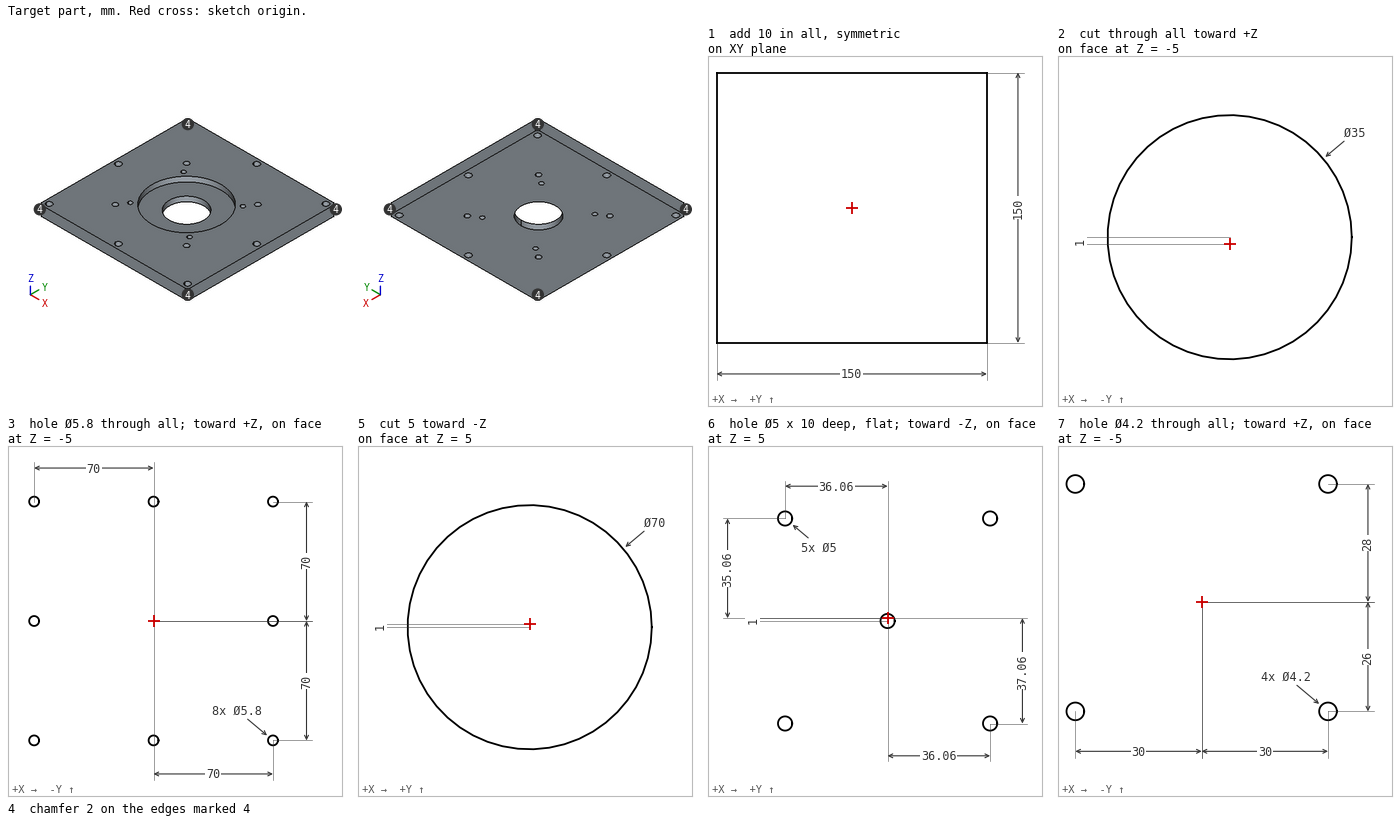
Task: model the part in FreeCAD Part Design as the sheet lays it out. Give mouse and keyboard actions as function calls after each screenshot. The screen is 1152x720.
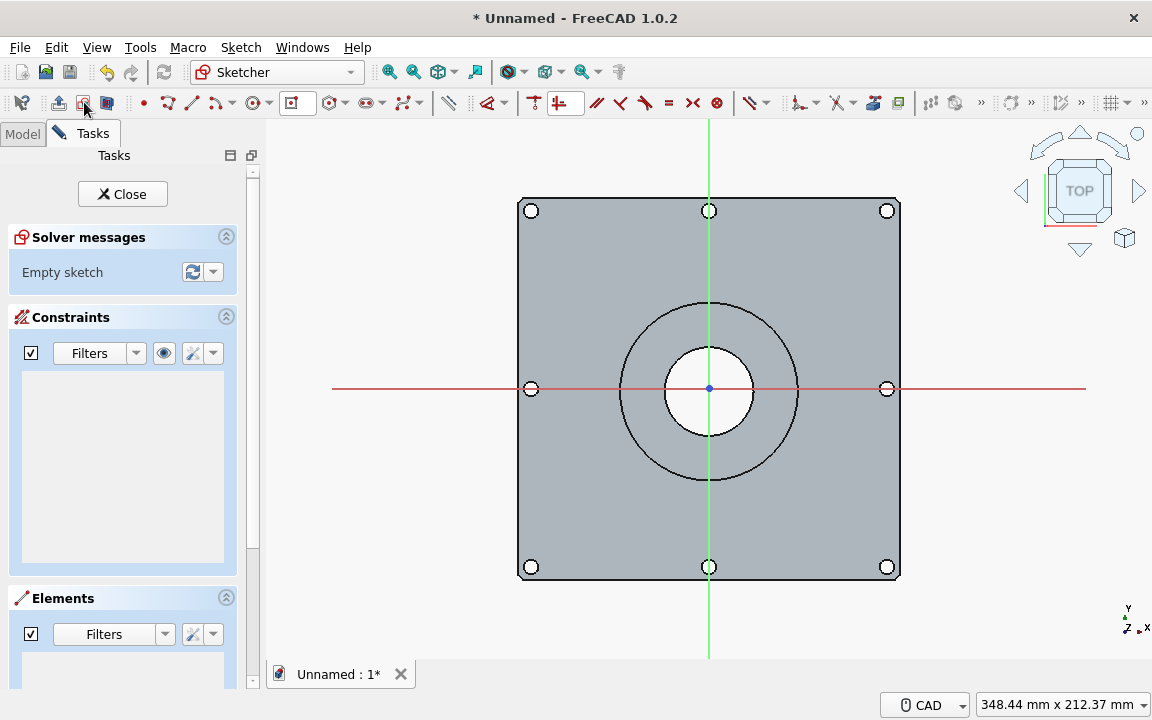
scroll(792, 395, up, 3)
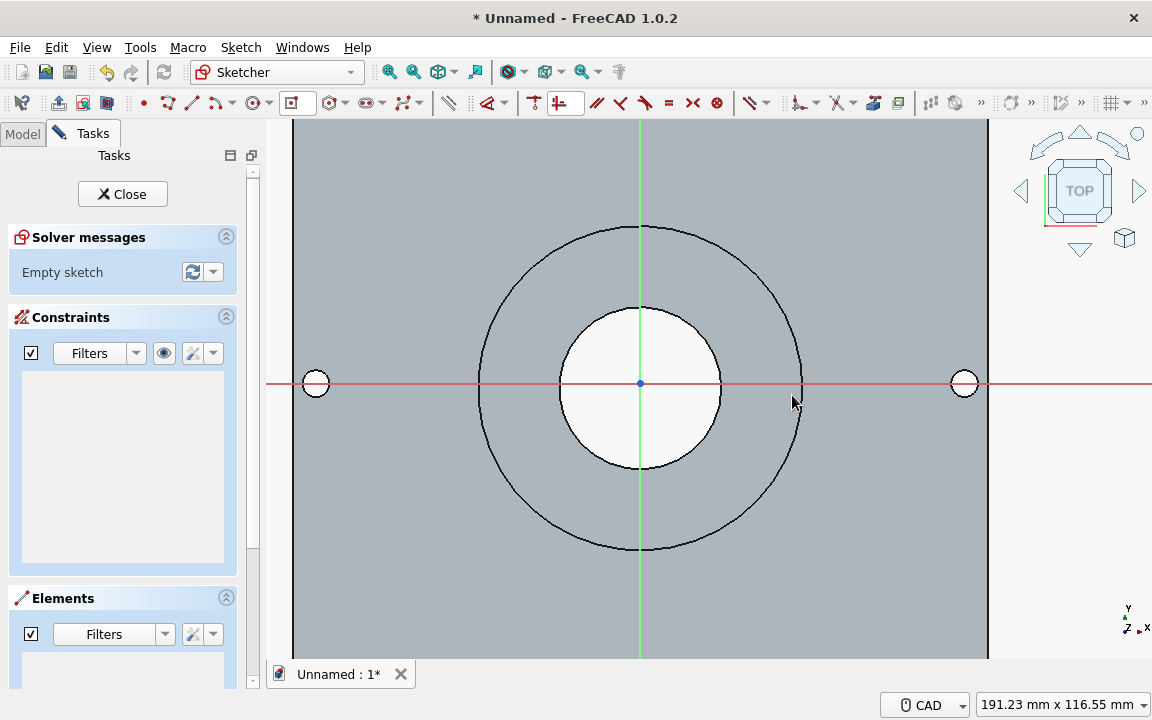
key(g)
key(c)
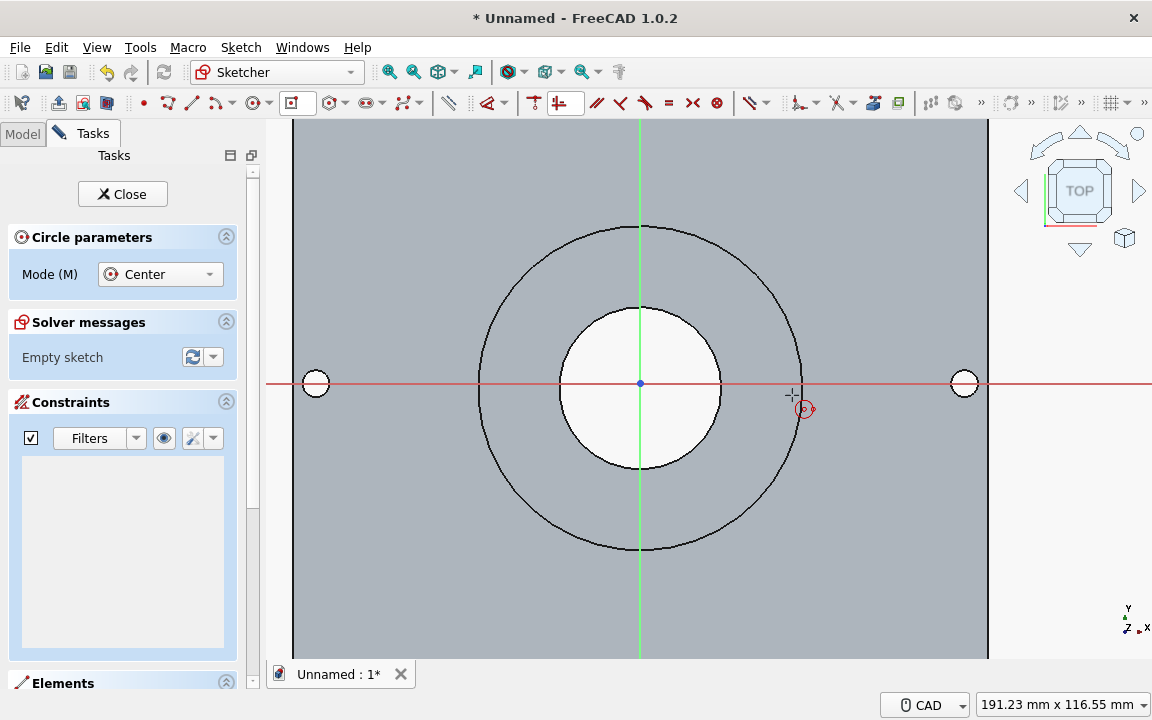
scroll(473, 221, up, 4)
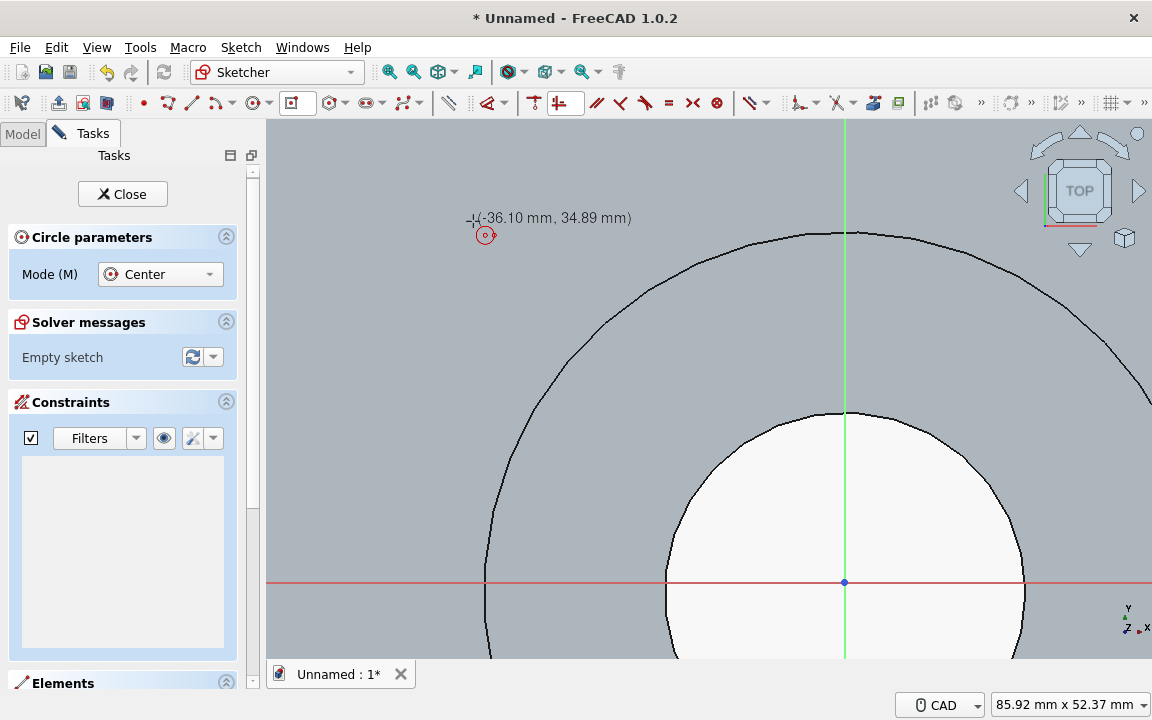
click(473, 221)
move(491, 203)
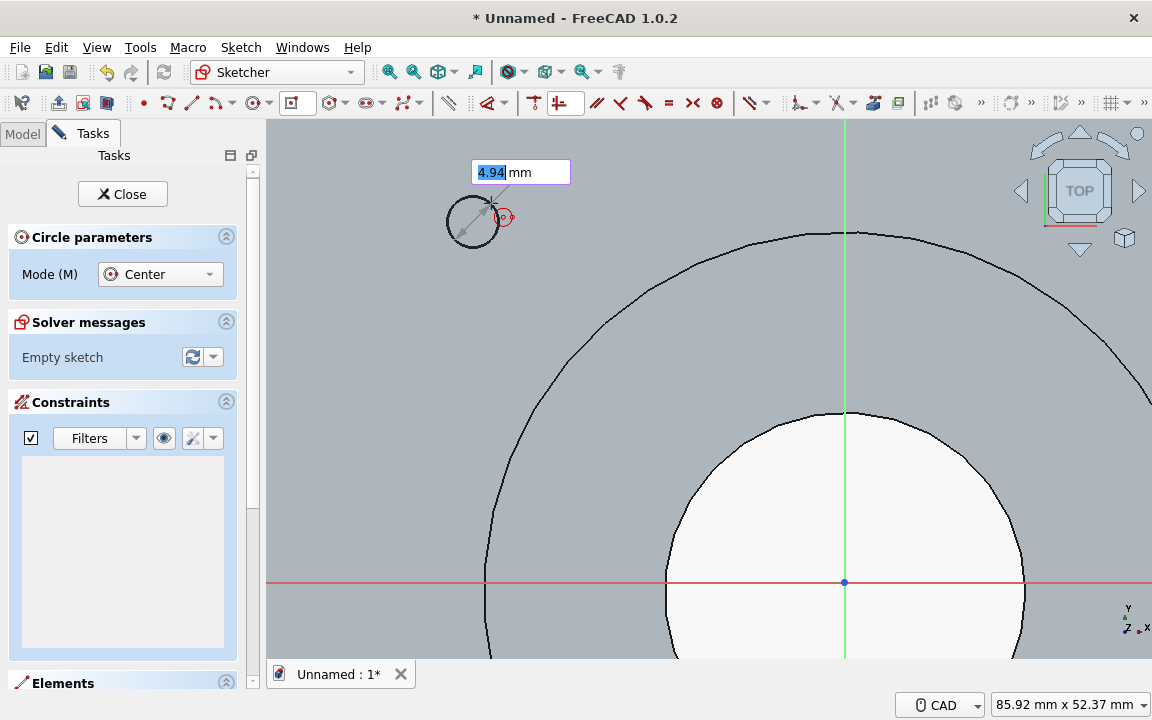
text(5)
key(Return)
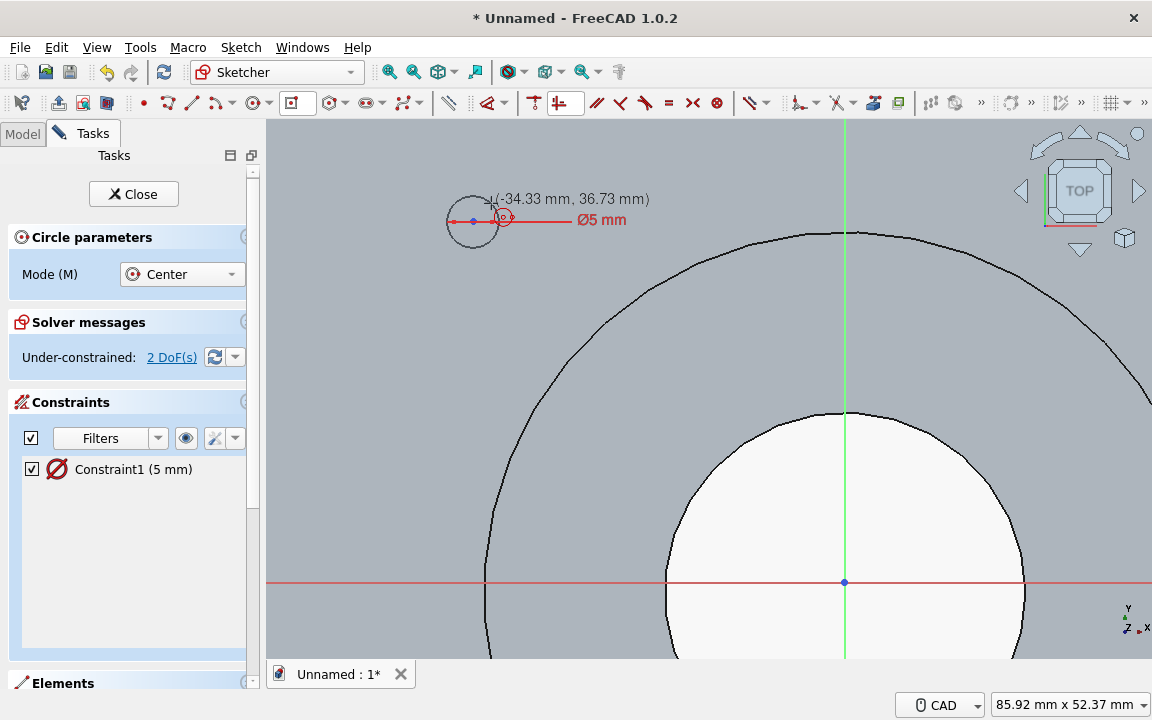
scroll(845, 593, up, 3)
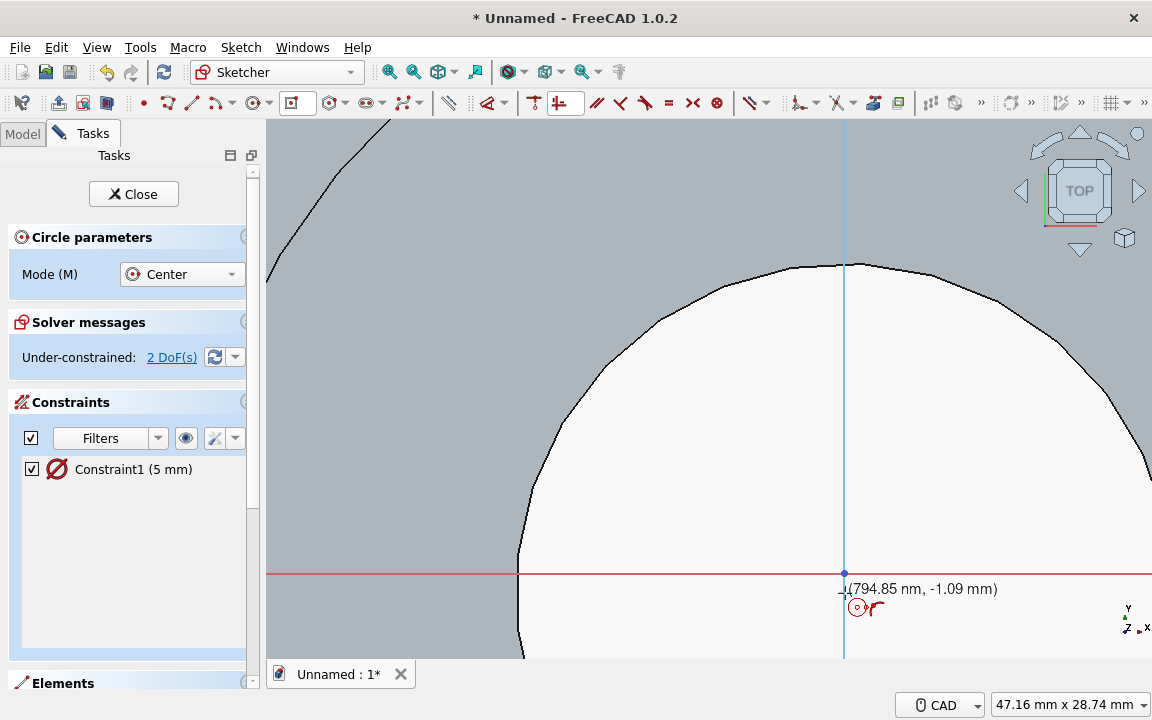
click(844, 592)
move(878, 559)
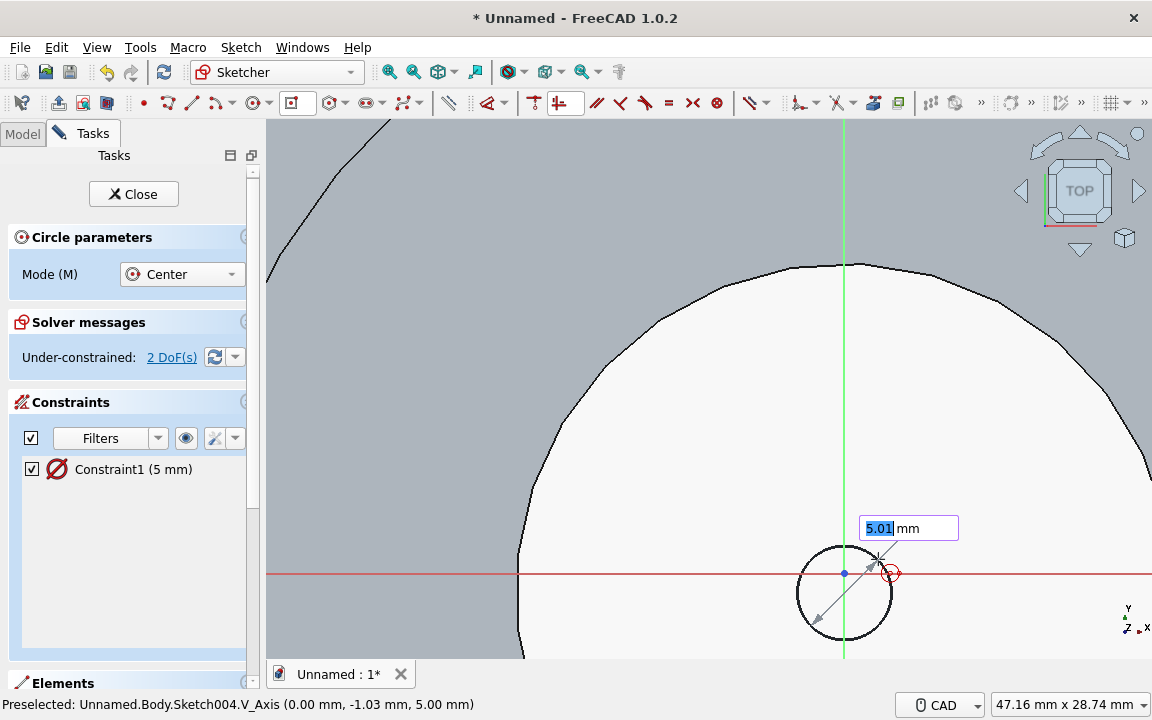
text(5)
key(Return)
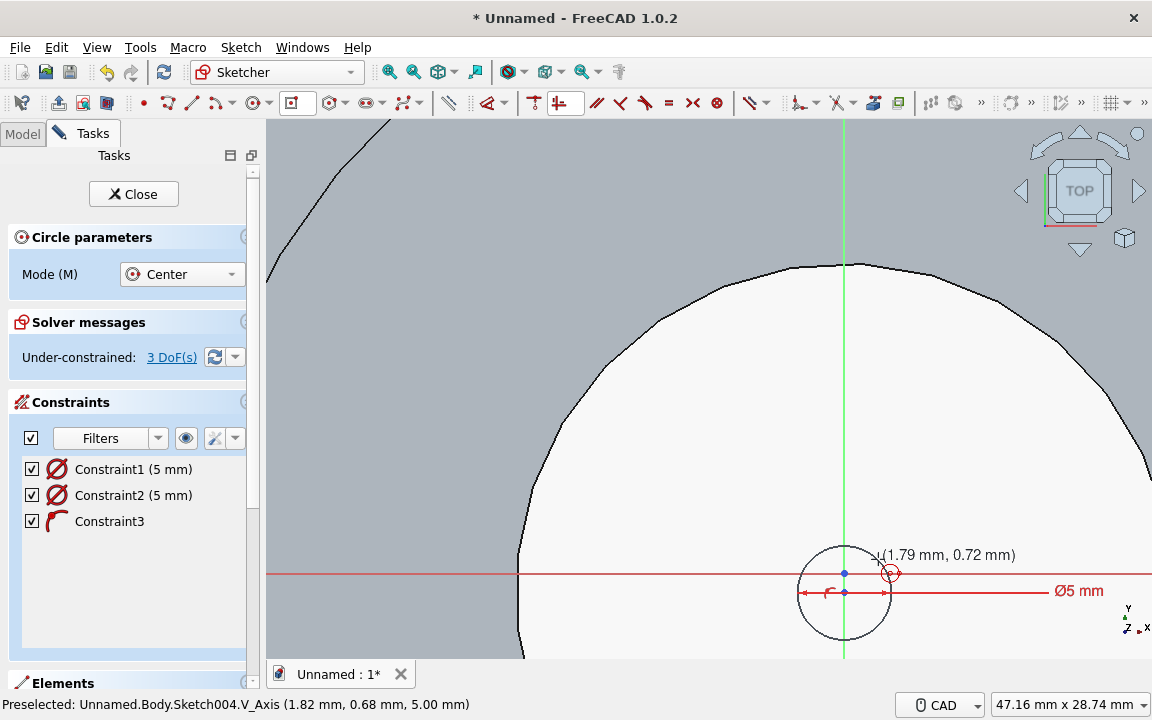
scroll(574, 322, down, 7)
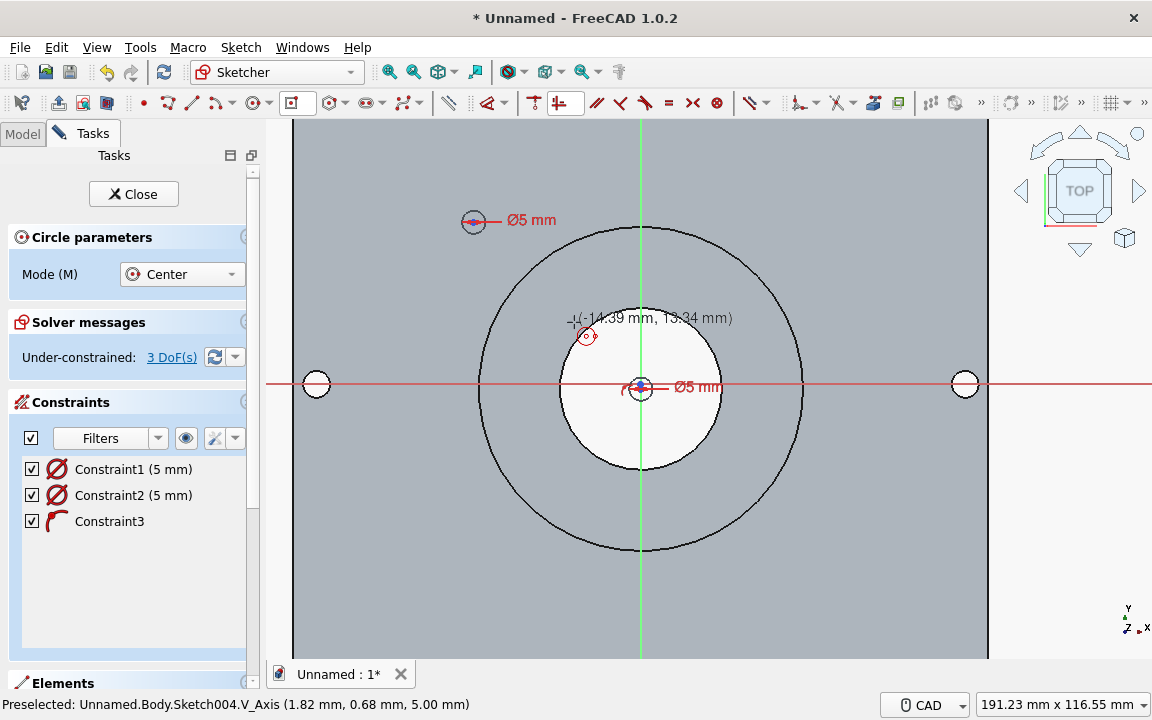
scroll(808, 556, up, 4)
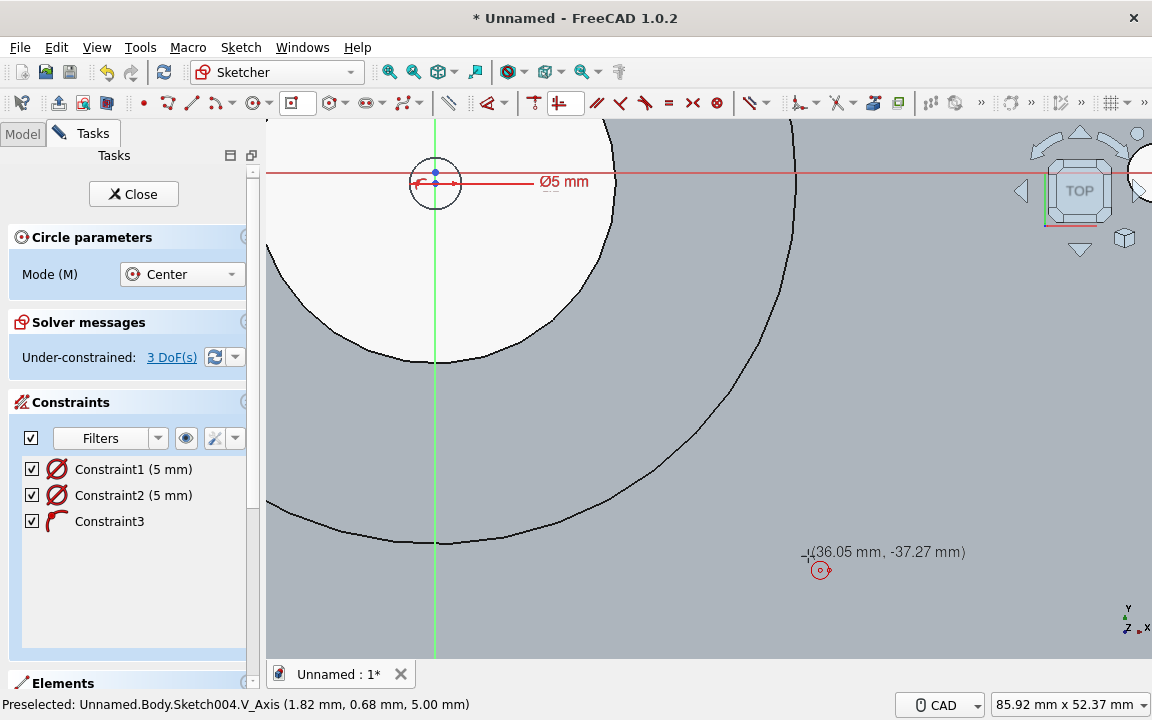
click(807, 555)
move(826, 537)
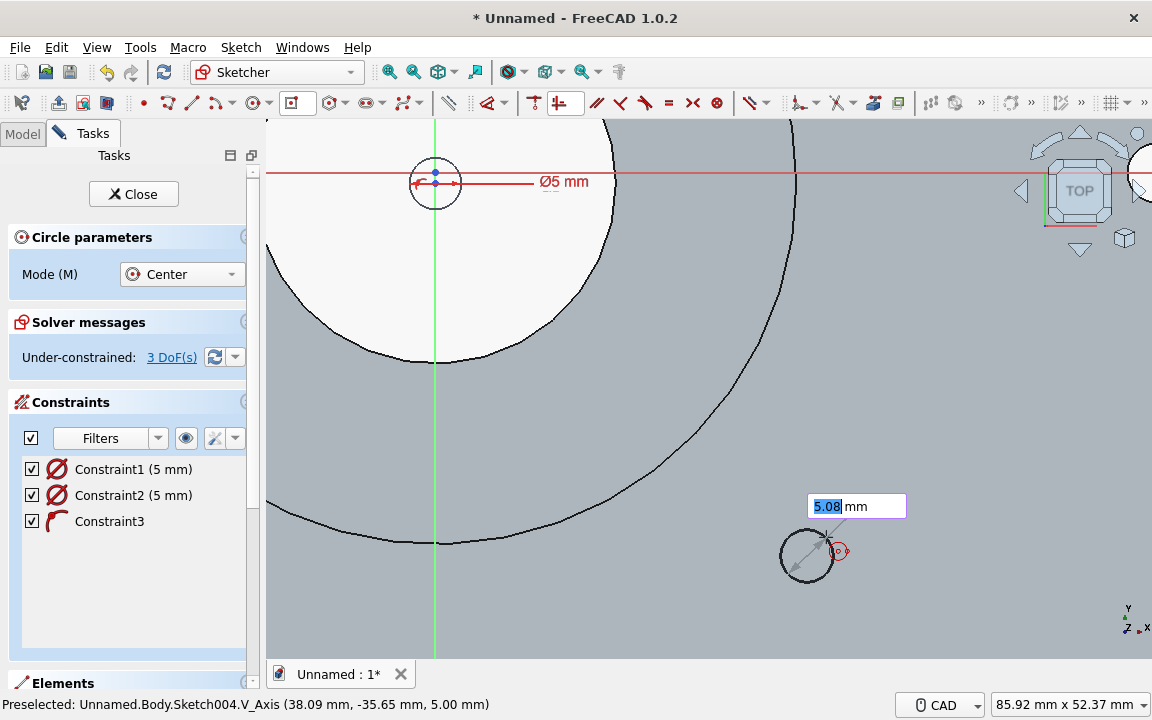
text(5)
key(Return)